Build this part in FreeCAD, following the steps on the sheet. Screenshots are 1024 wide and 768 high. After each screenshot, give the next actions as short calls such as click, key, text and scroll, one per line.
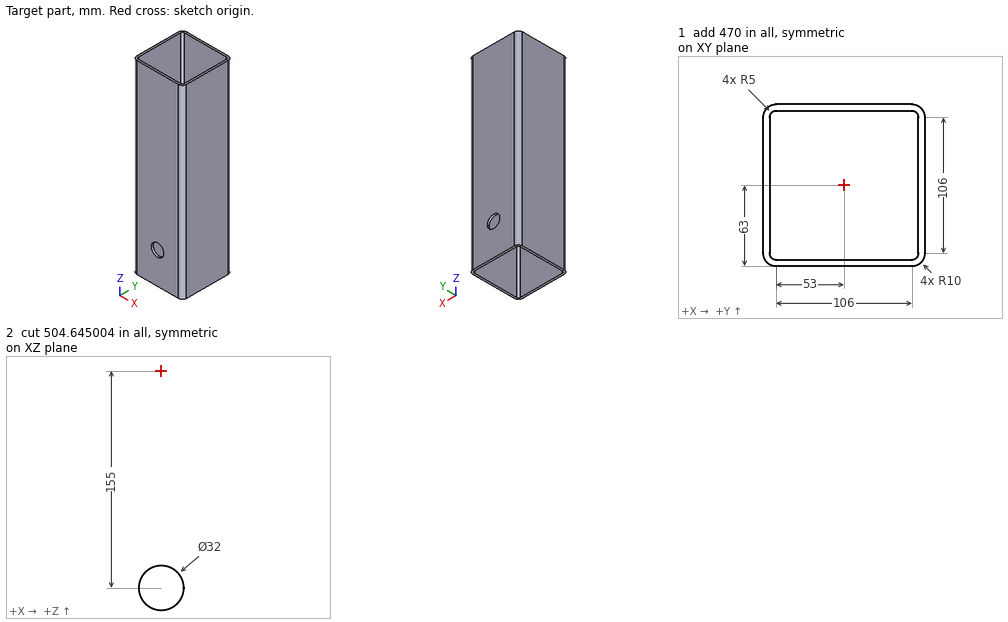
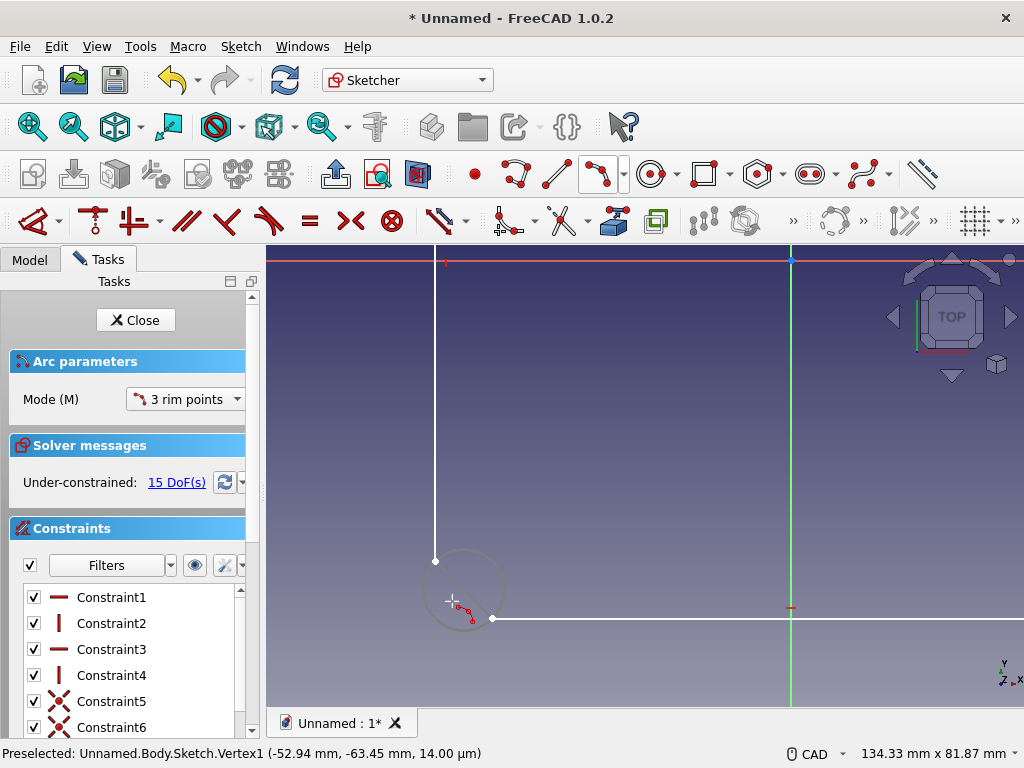
click(452, 600)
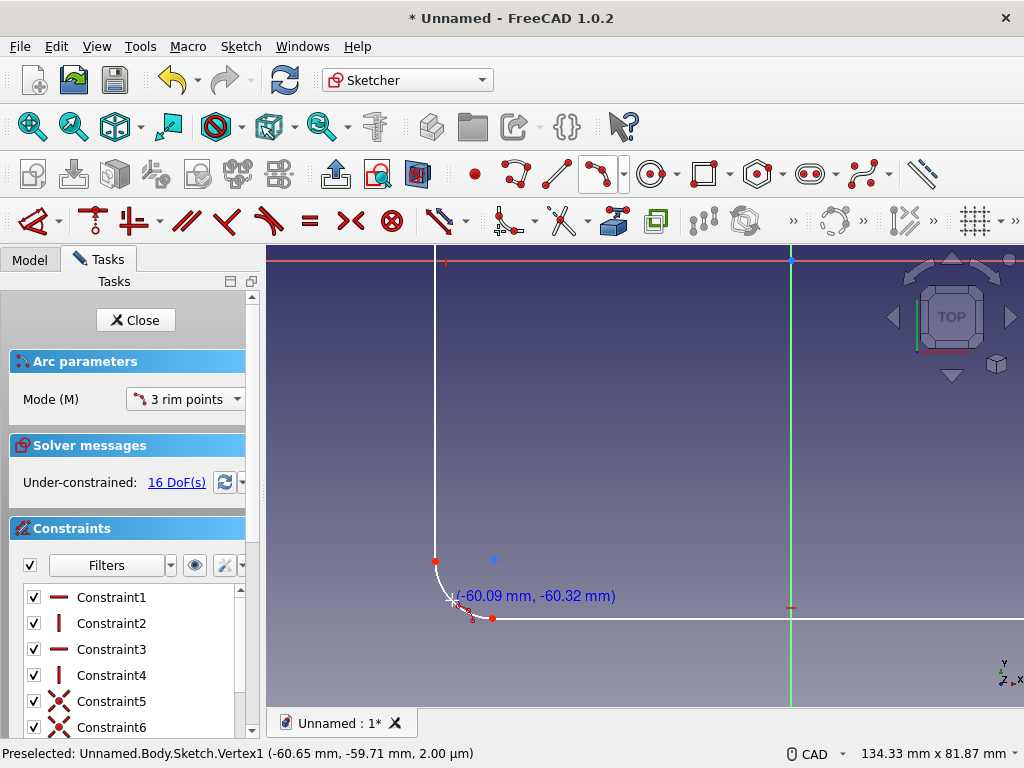
click(557, 174)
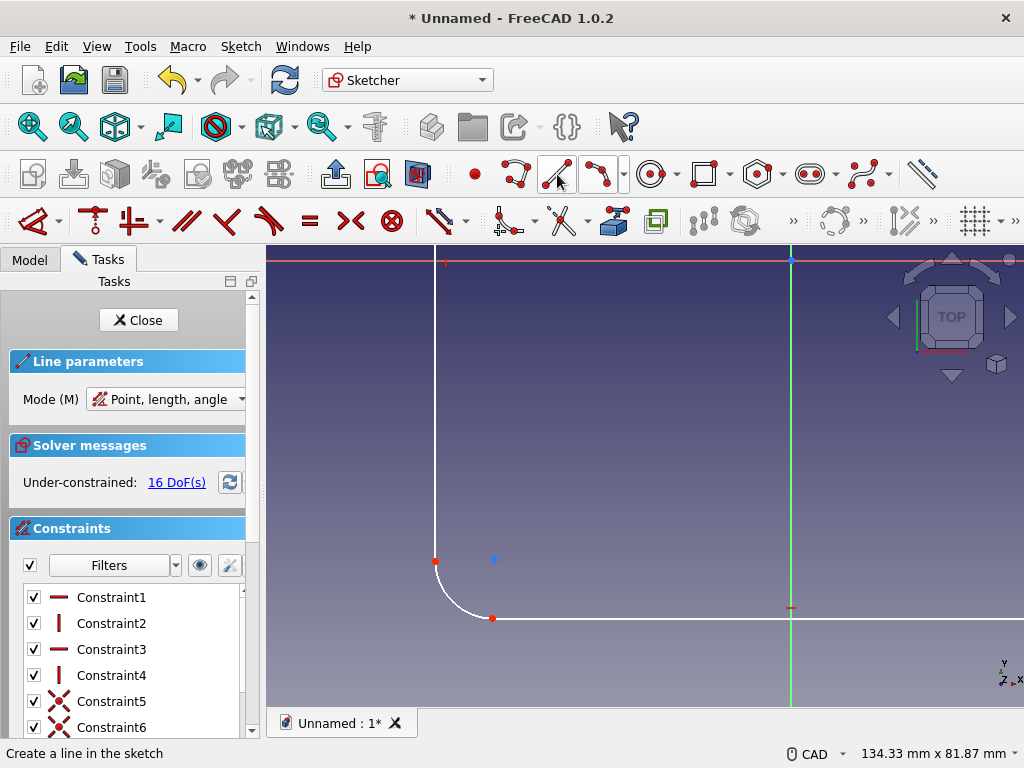
scroll(452, 601, down, 5)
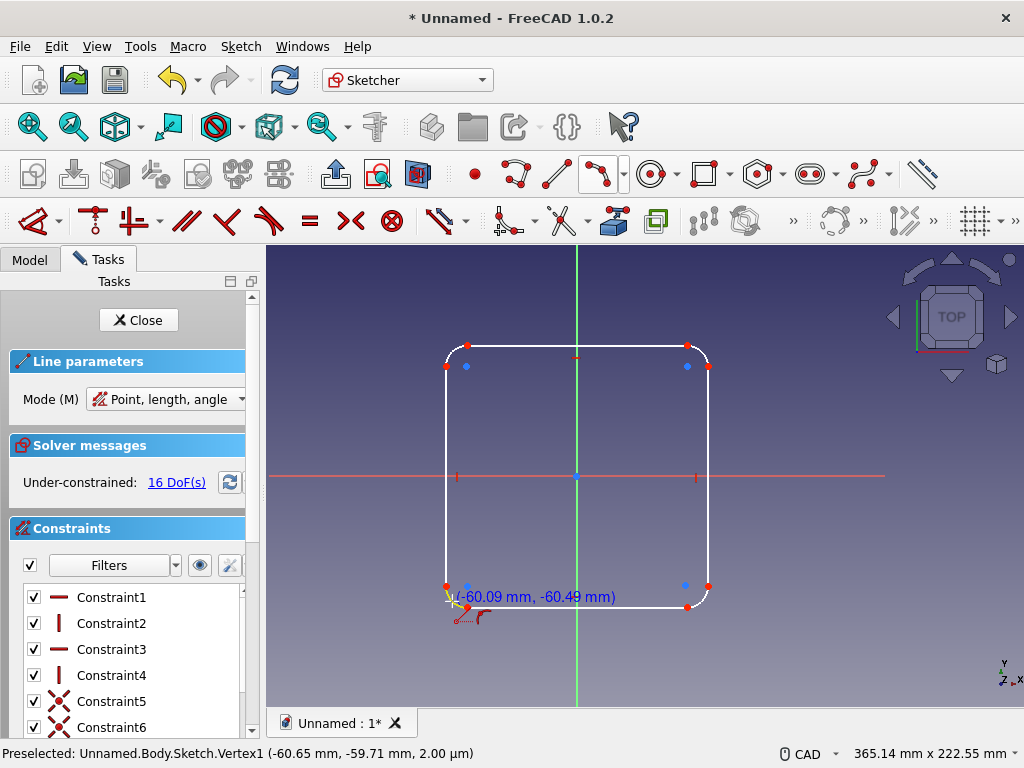
scroll(687, 597, up, 3)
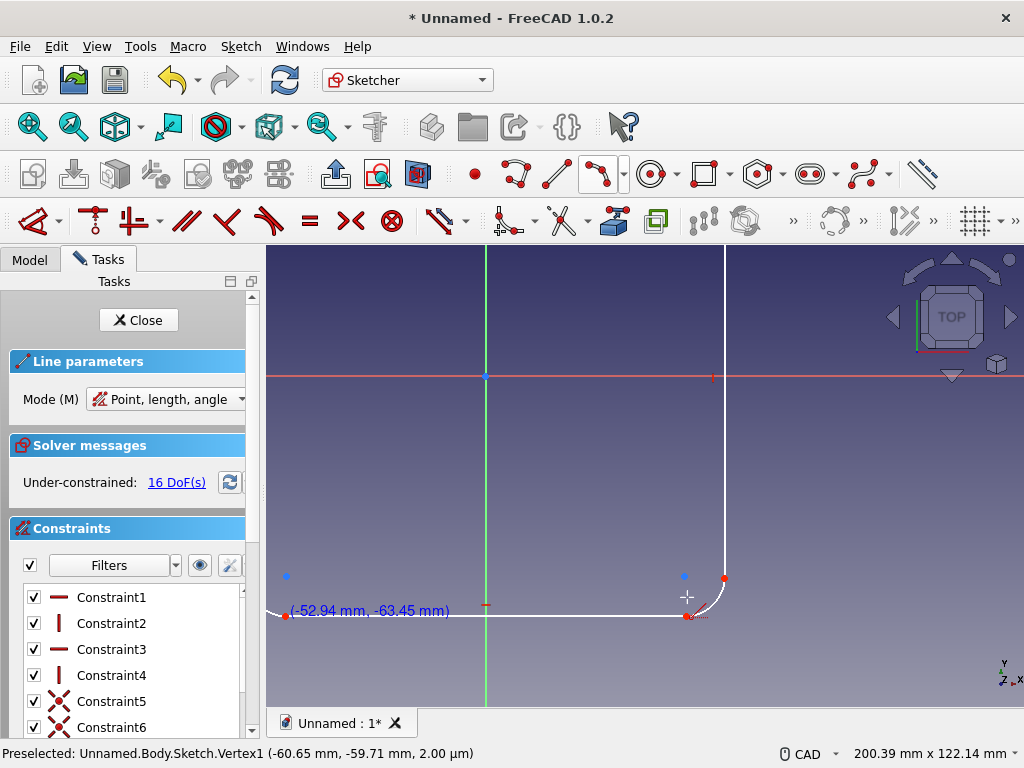
click(686, 596)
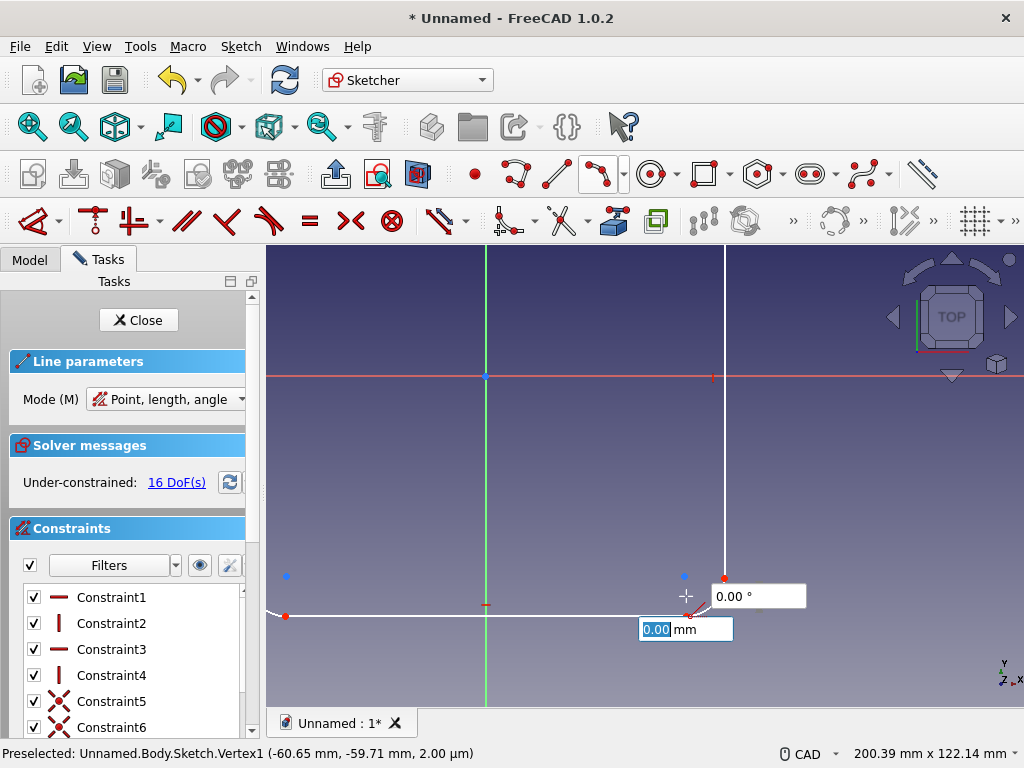
scroll(687, 597, down, 3)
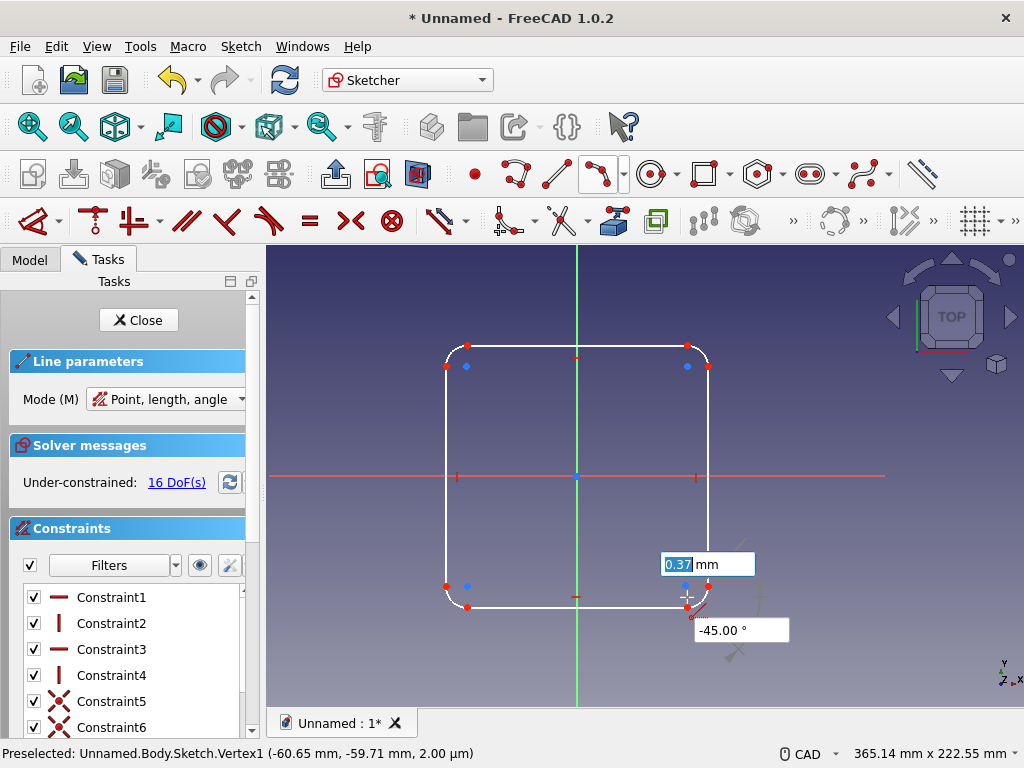
scroll(467, 597, up, 3)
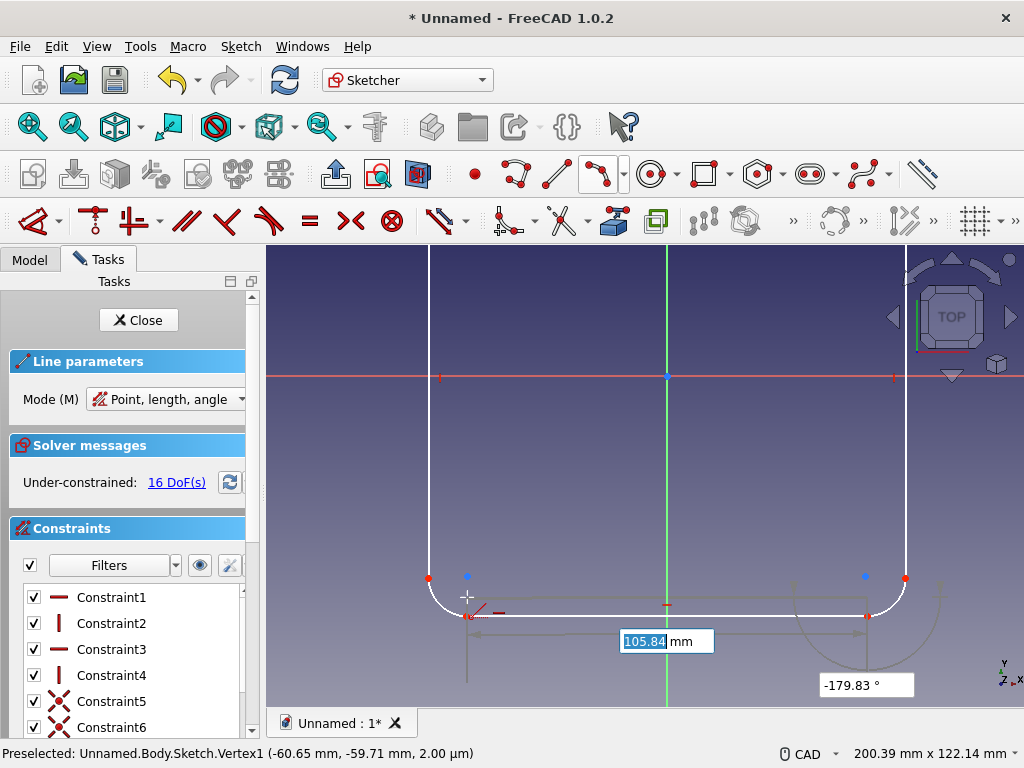
click(467, 596)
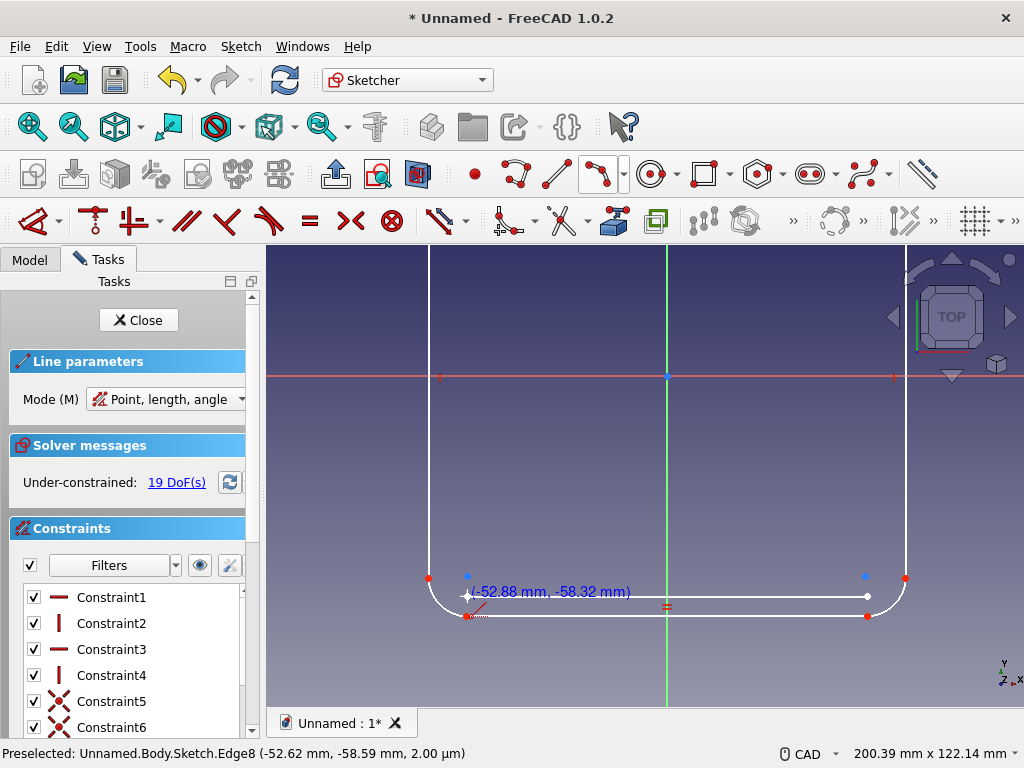
click(448, 577)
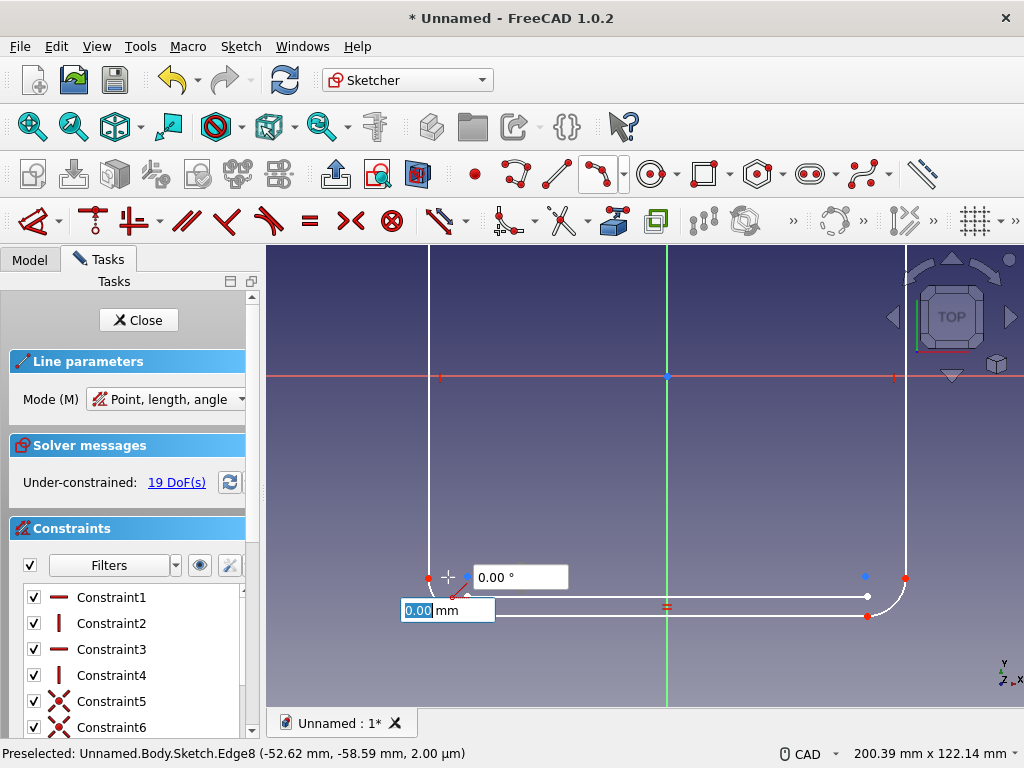
scroll(466, 597, down, 3)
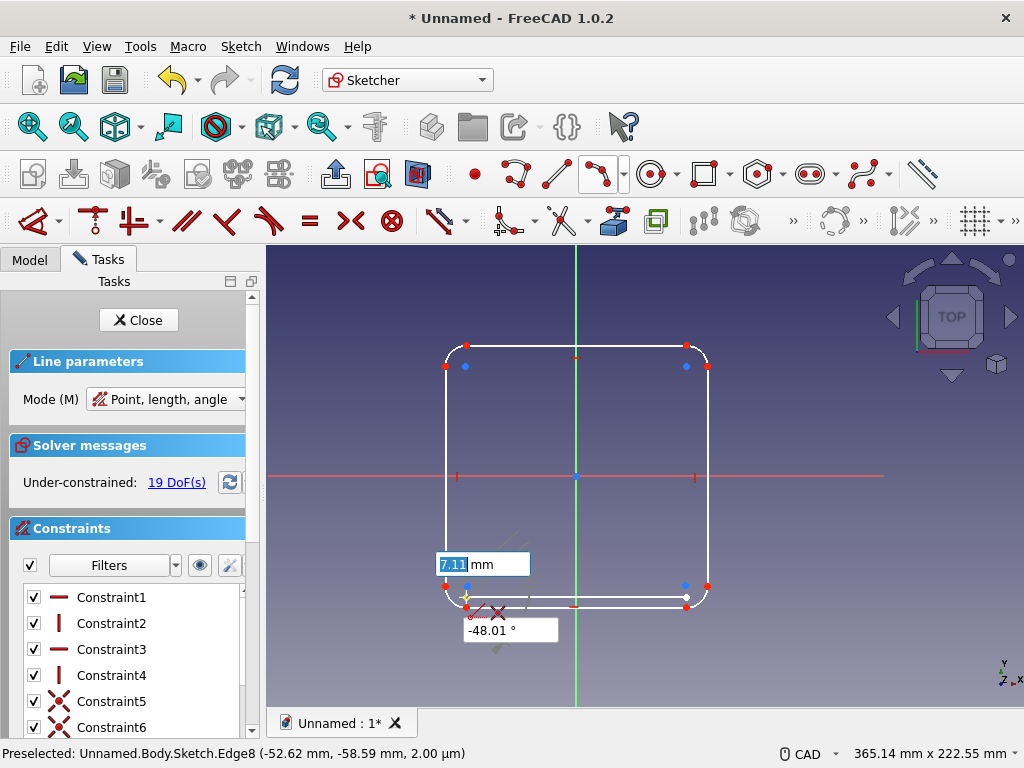
scroll(456, 366, up, 3)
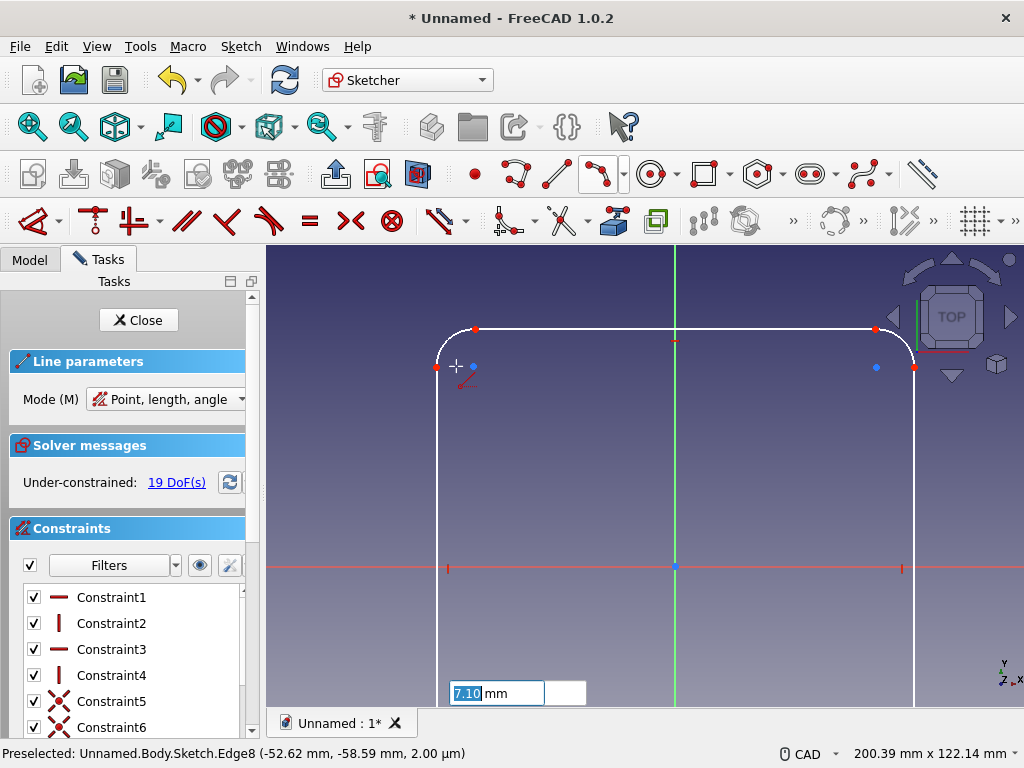
click(456, 366)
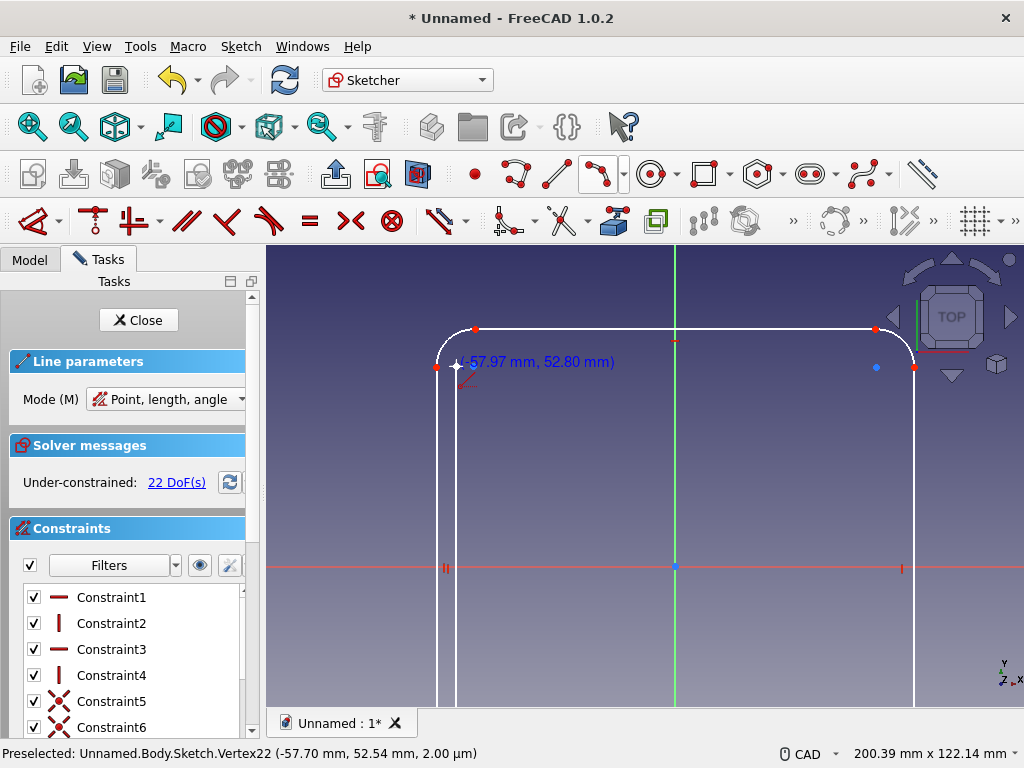
click(475, 347)